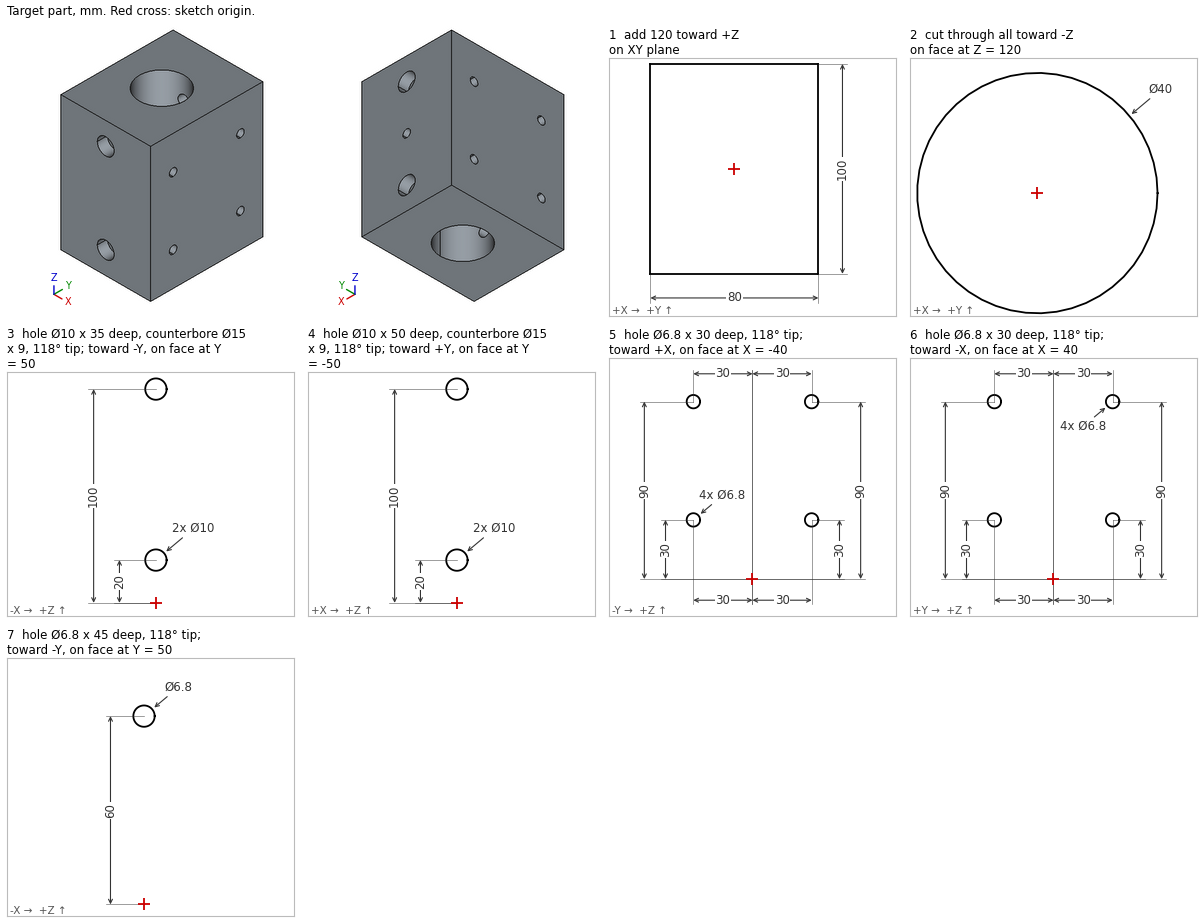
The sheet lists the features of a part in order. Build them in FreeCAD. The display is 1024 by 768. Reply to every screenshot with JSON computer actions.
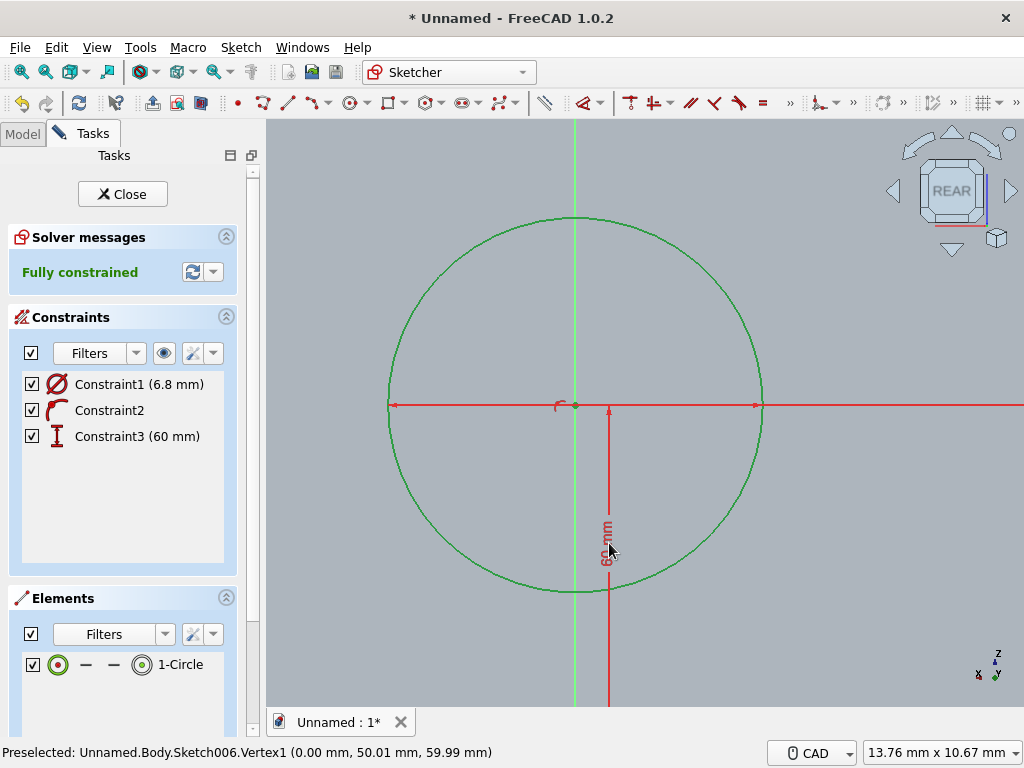
{"action": "left_click", "coordinate": [123, 194]}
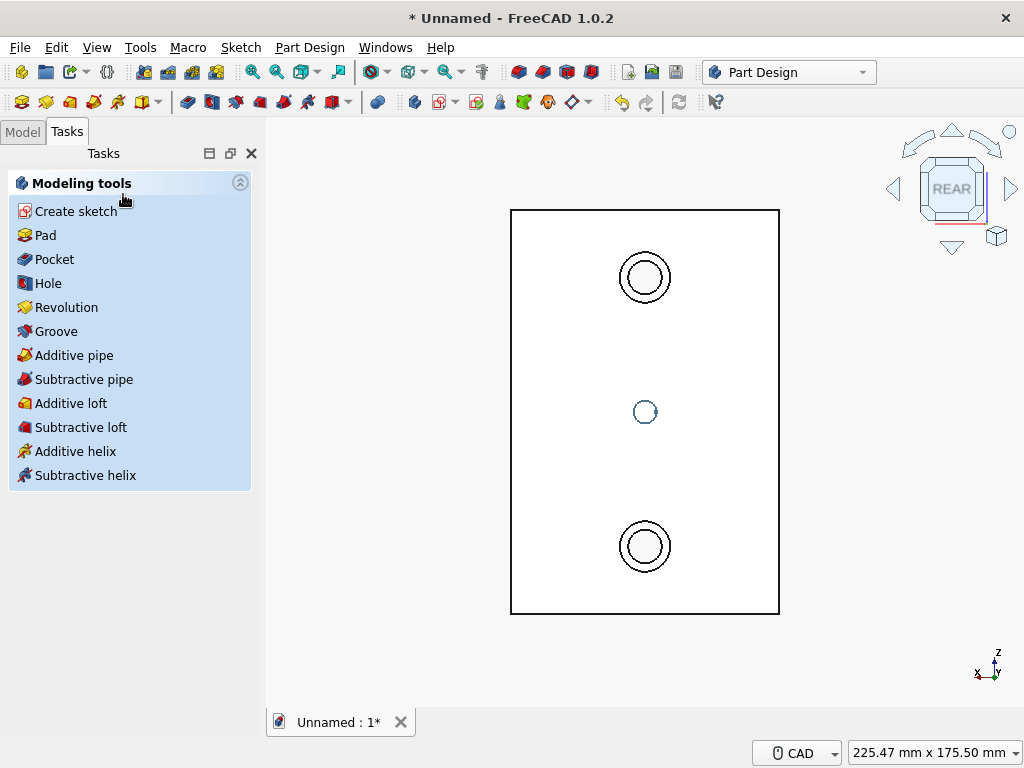
{"action": "left_click", "coordinate": [212, 102]}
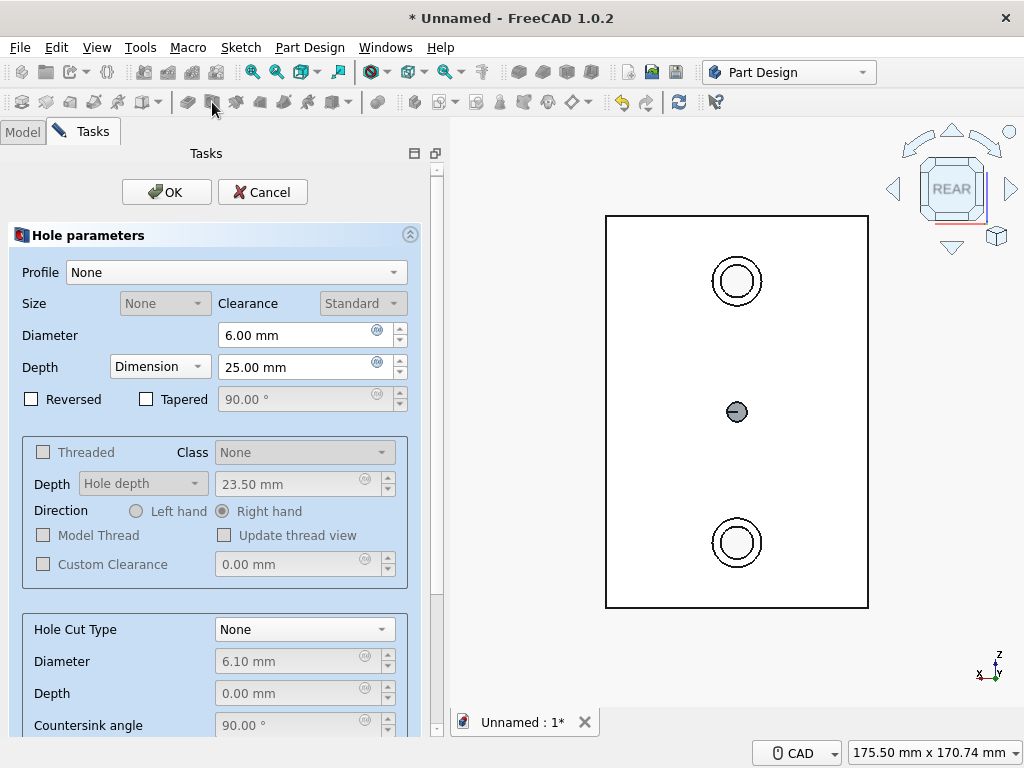
{"action": "triple_click", "coordinate": [305, 335]}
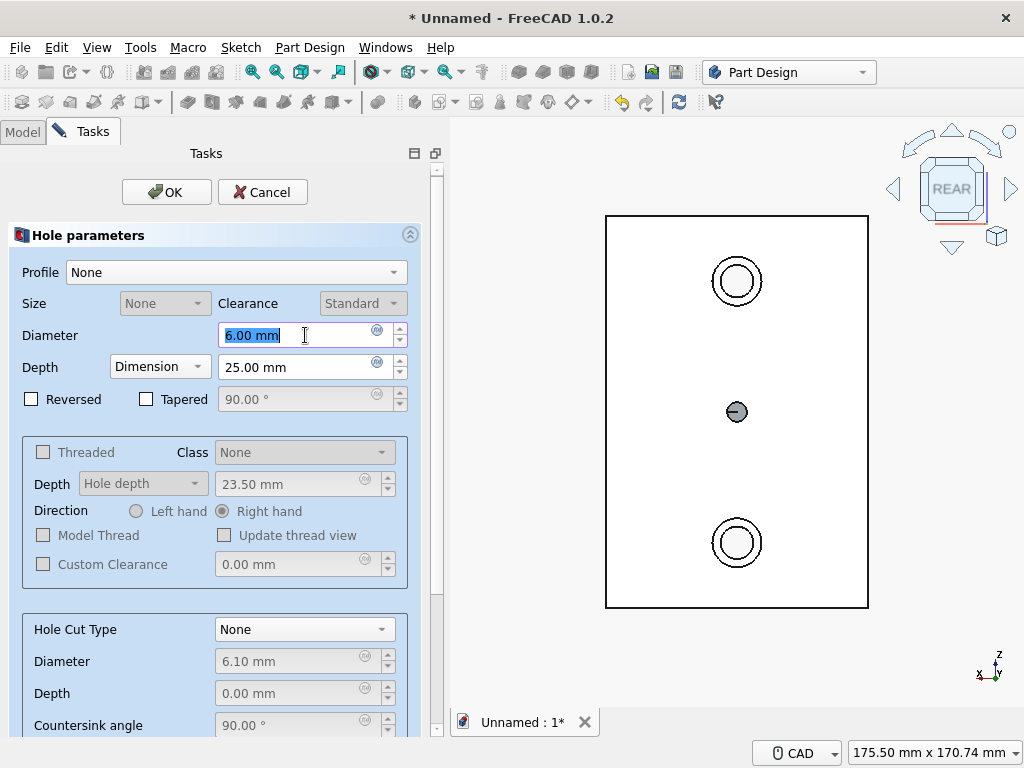
{"action": "type", "text": "6.8"}
{"action": "key", "text": "Tab"}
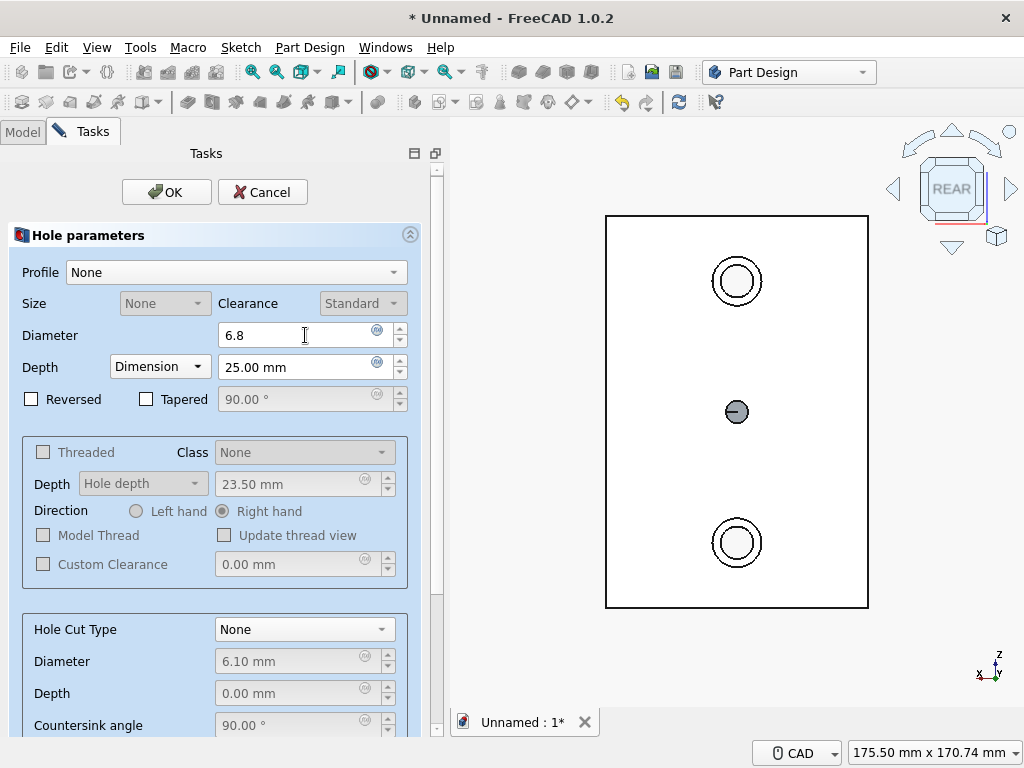
{"action": "triple_click", "coordinate": [305, 367]}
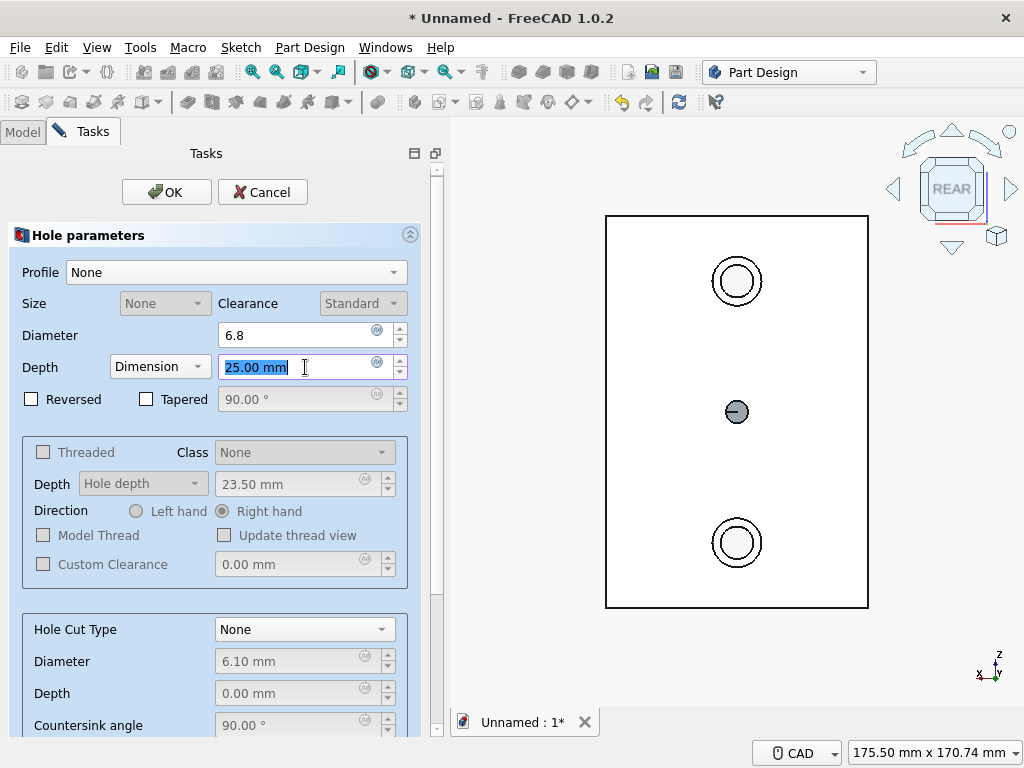
{"action": "type", "text": "45"}
{"action": "key", "text": "Tab"}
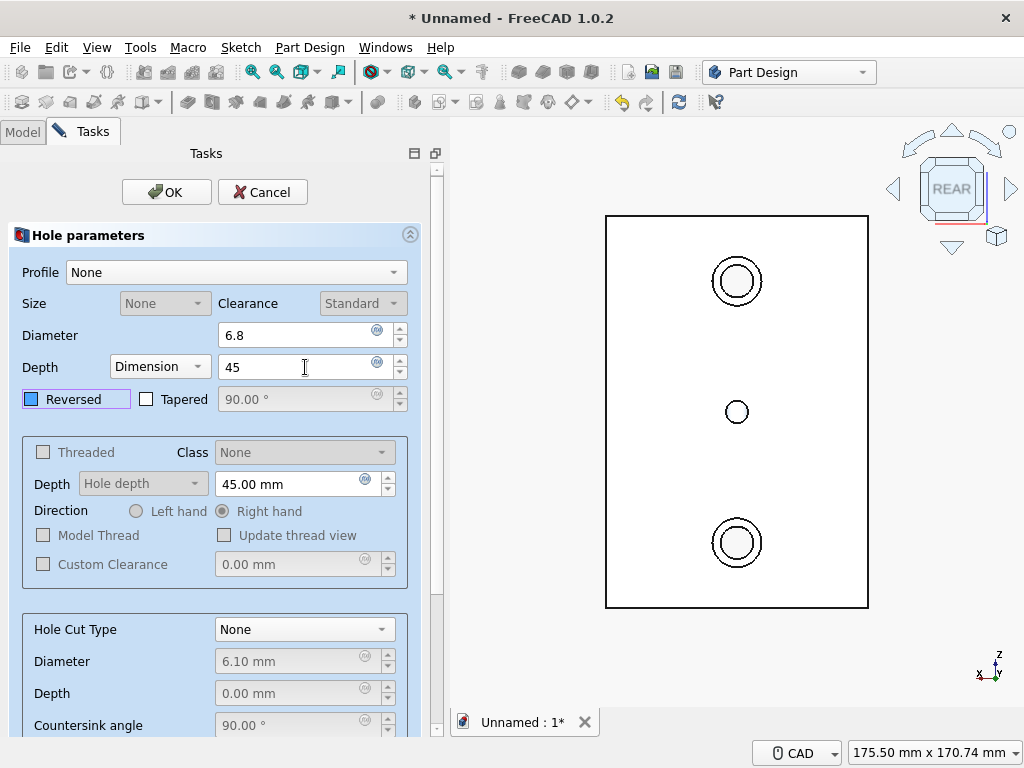
{"action": "left_click", "coordinate": [167, 192]}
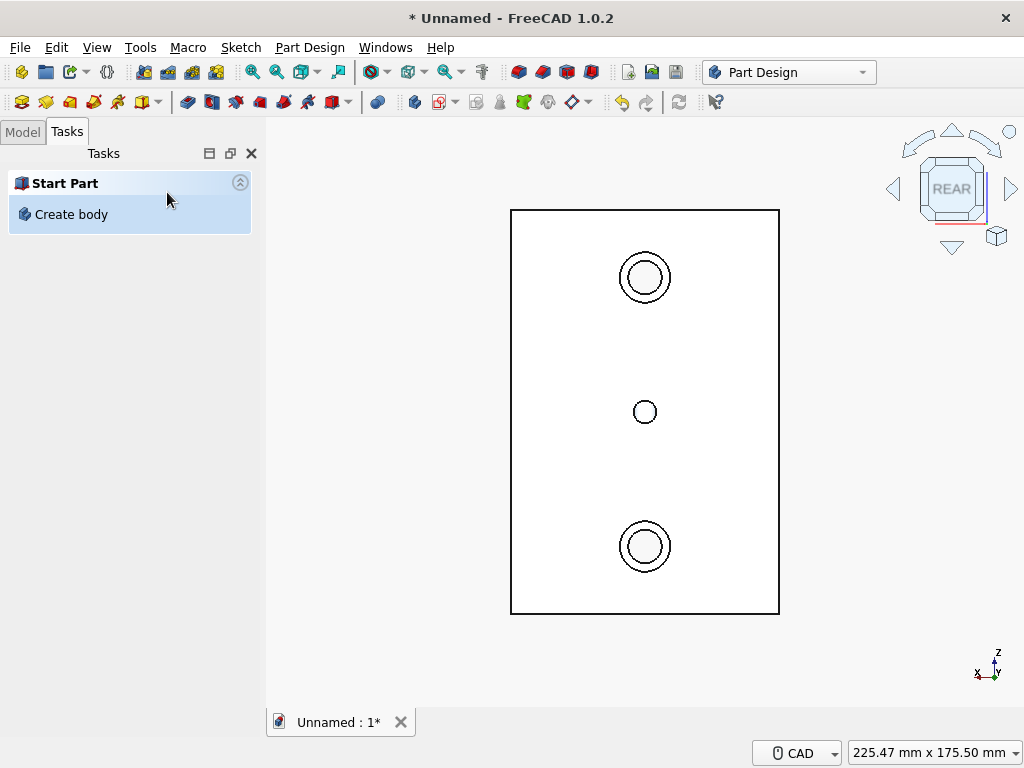
{"action": "key", "text": "0"}